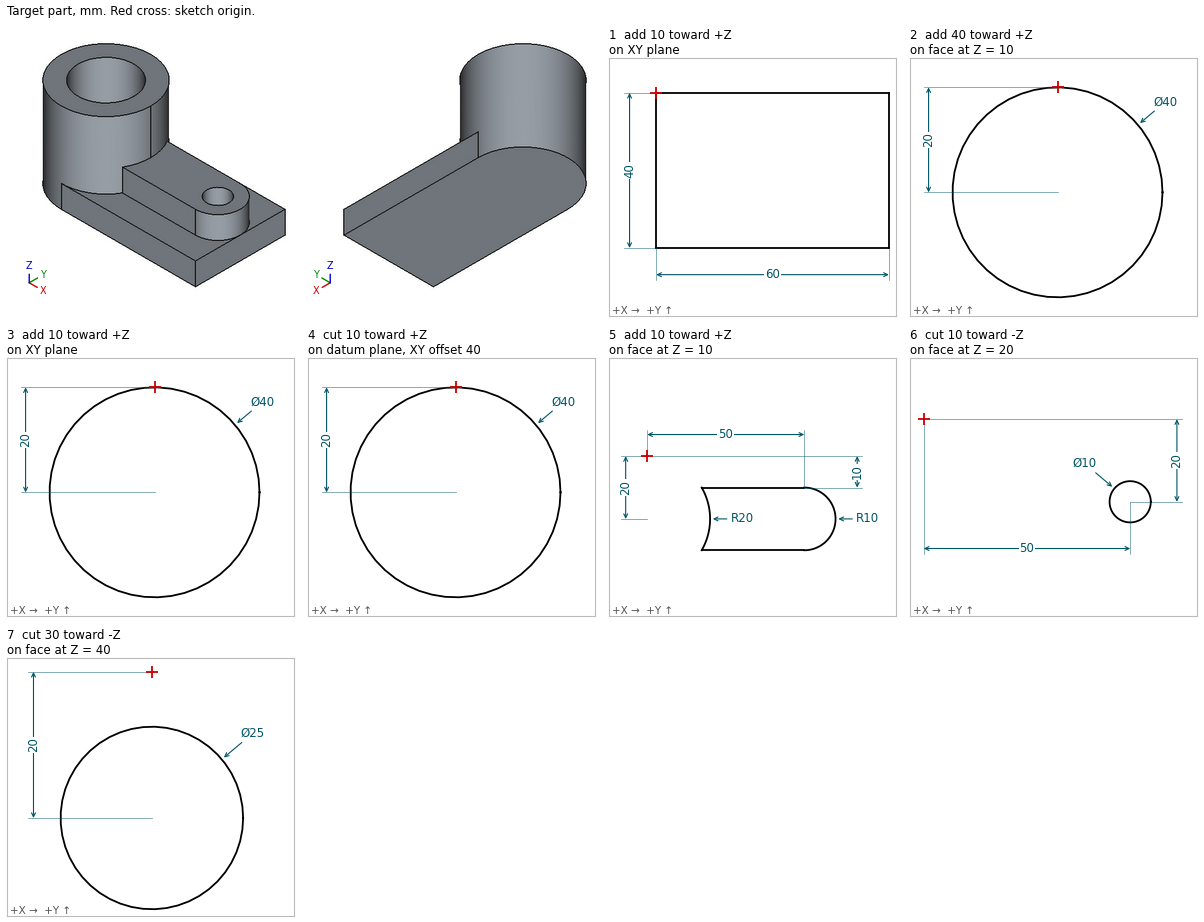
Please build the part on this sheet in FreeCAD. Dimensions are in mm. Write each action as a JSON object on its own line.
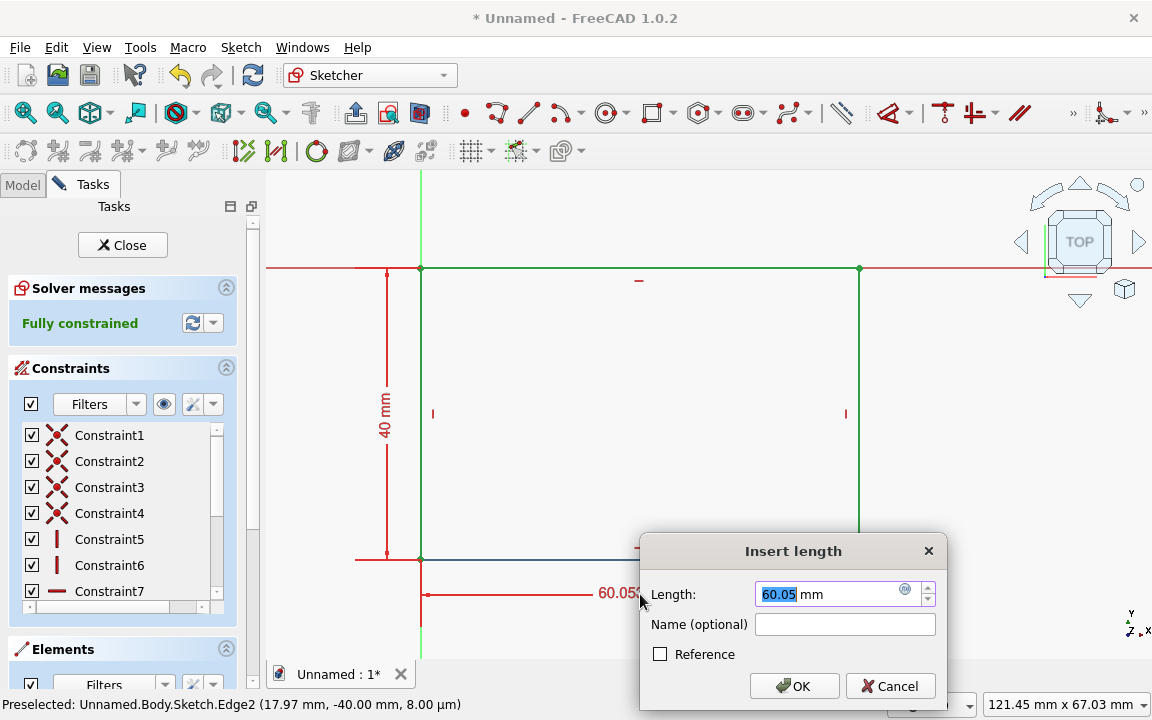
{"action": "type", "text": "60"}
{"action": "key", "text": "Return"}
{"action": "key", "text": "Escape"}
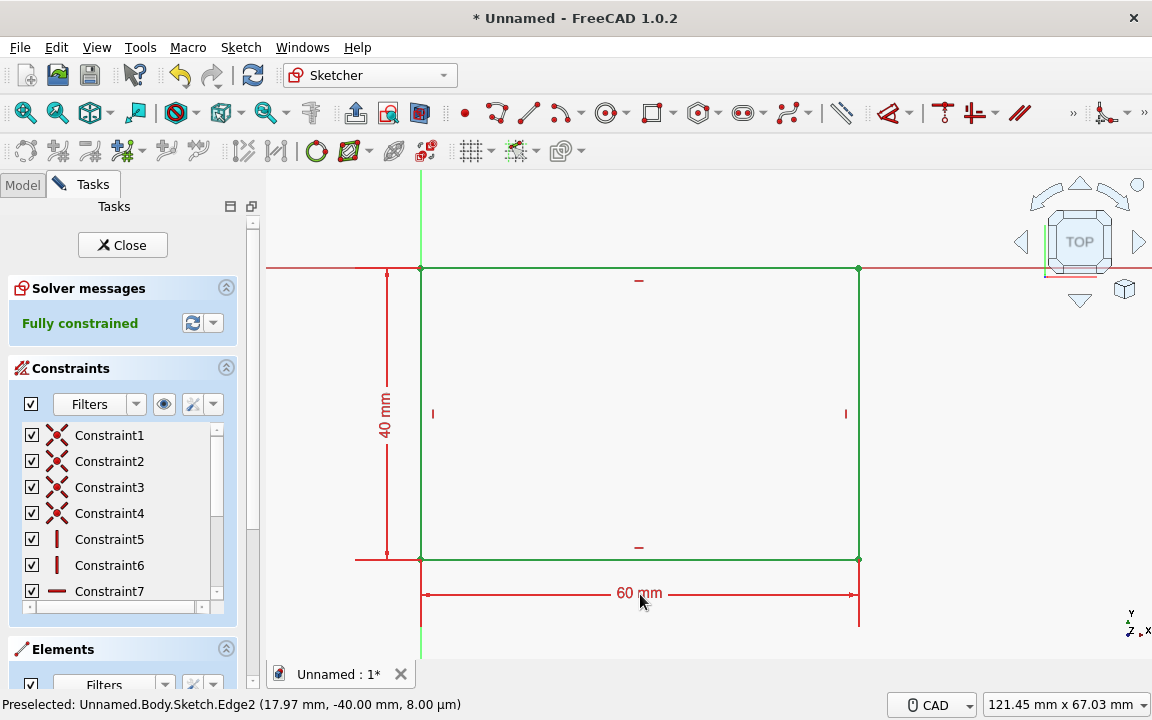
{"action": "left_click", "coordinate": [123, 245]}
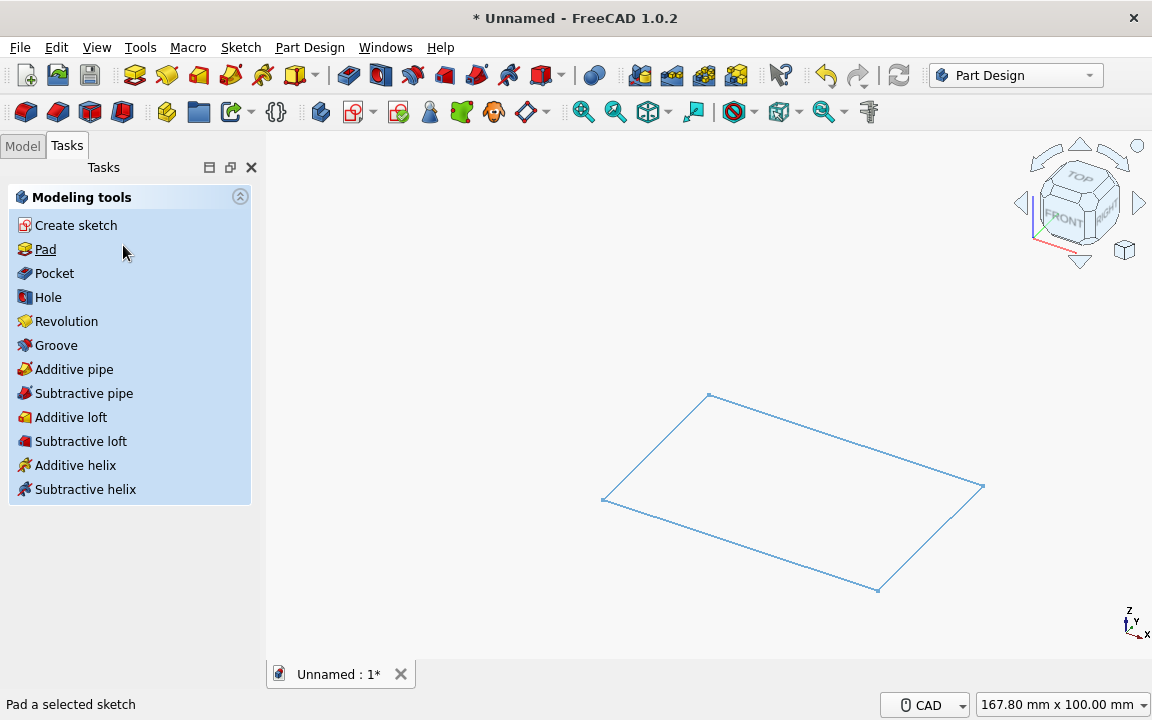
{"action": "left_click", "coordinate": [136, 76]}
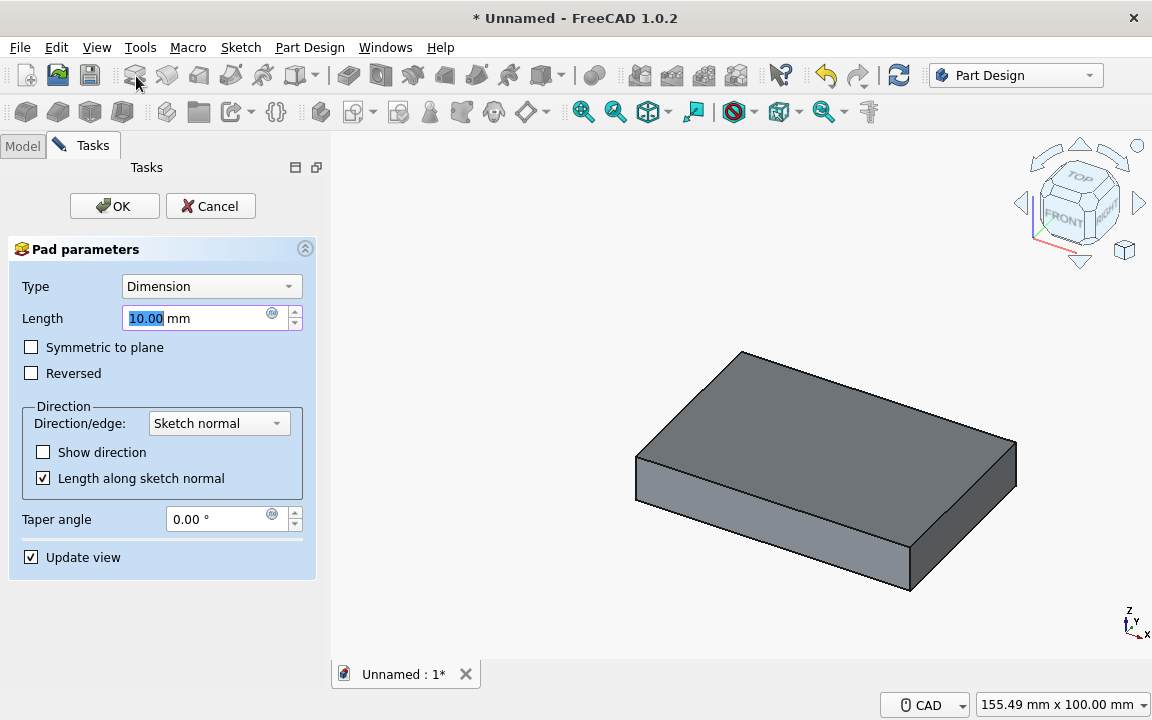
{"action": "type", "text": "10"}
{"action": "key", "text": "Tab"}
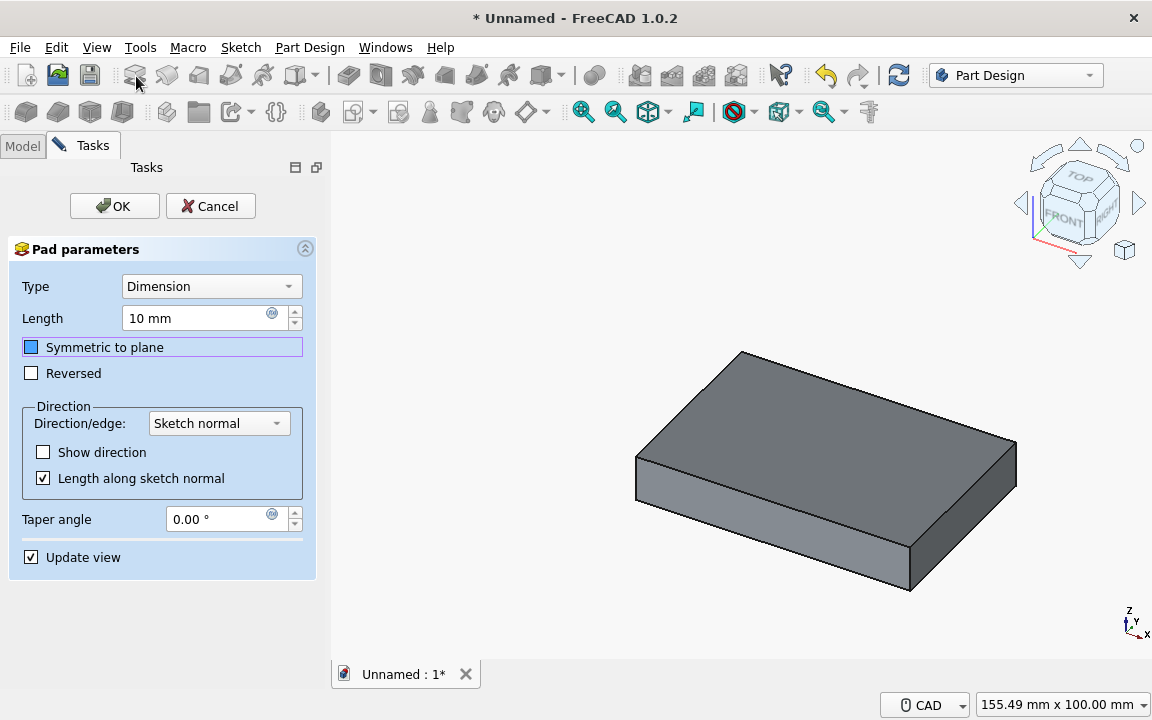
{"action": "left_click", "coordinate": [115, 206]}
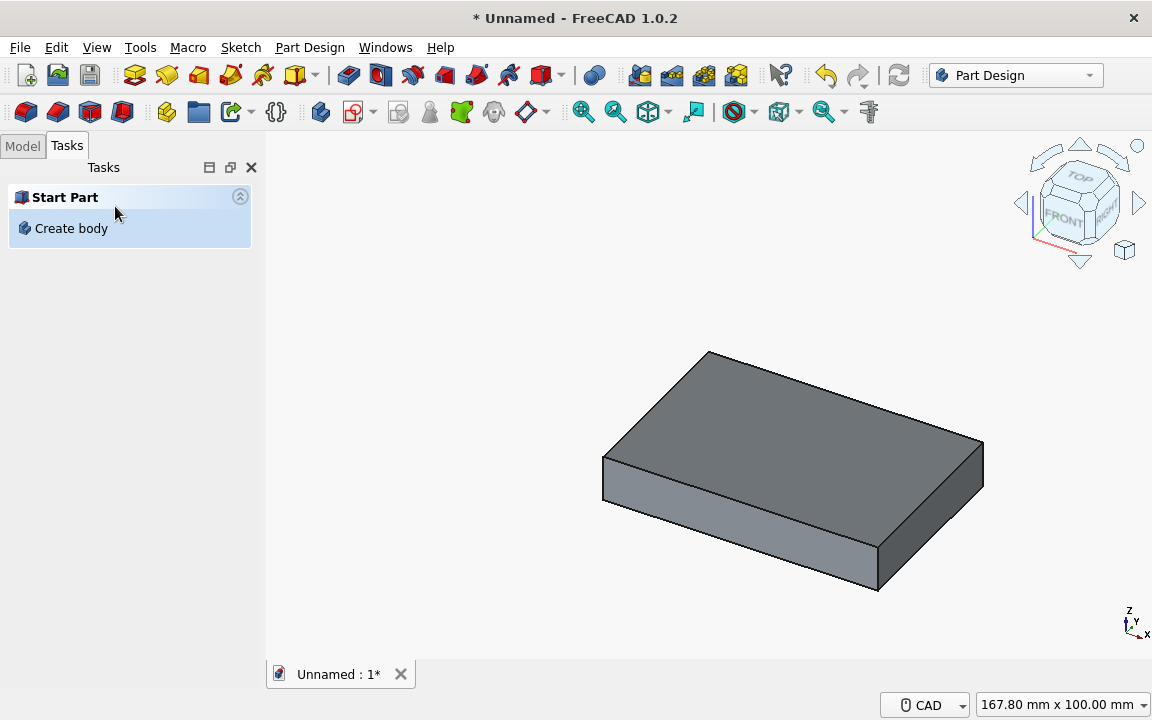
{"action": "left_click", "coordinate": [833, 462]}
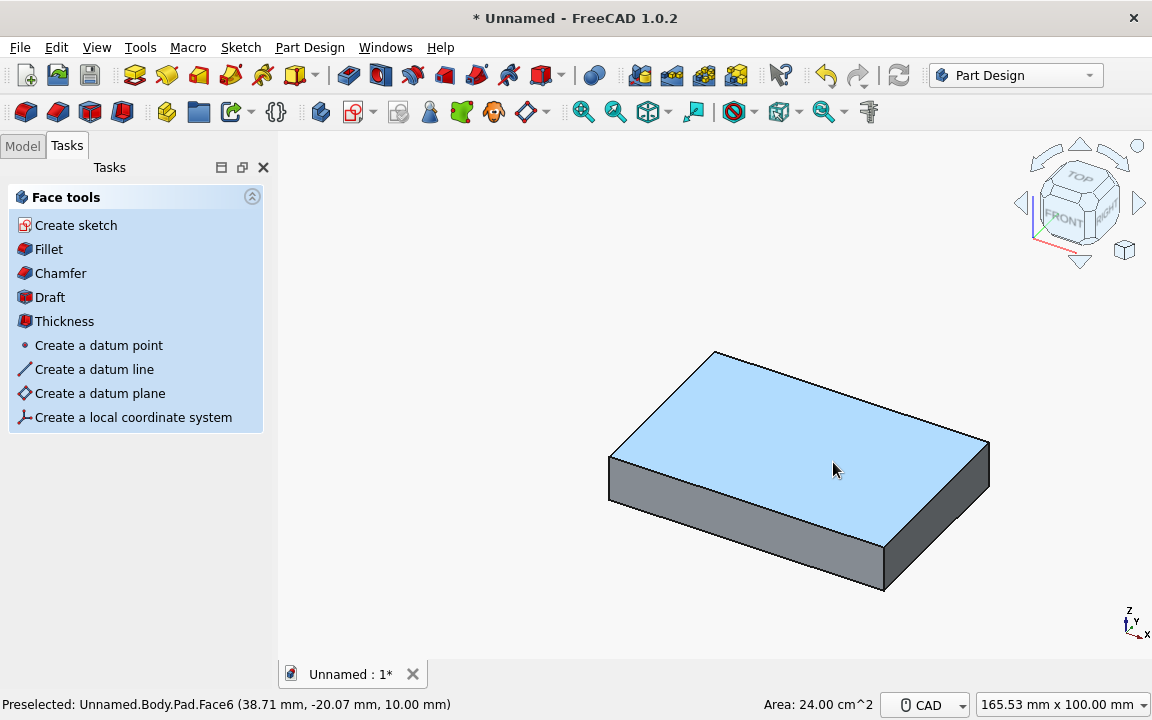
{"action": "left_click", "coordinate": [354, 112]}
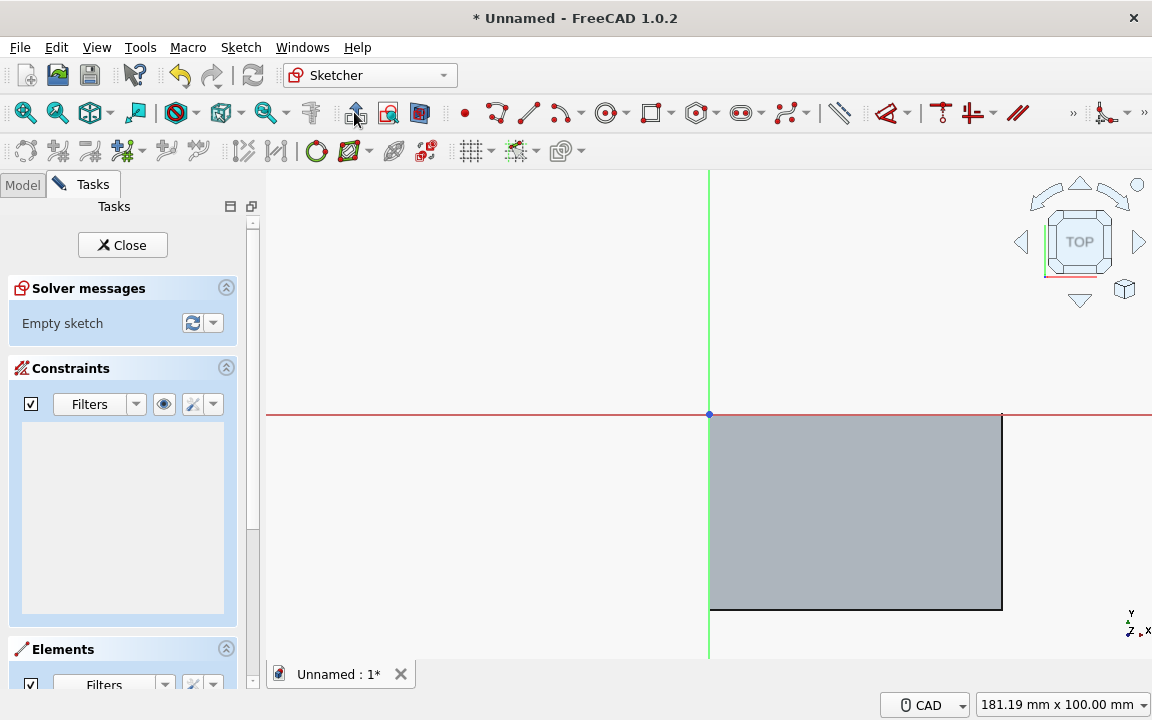
{"action": "scroll", "coordinate": [848, 631], "scroll_direction": "up", "scroll_amount": 2}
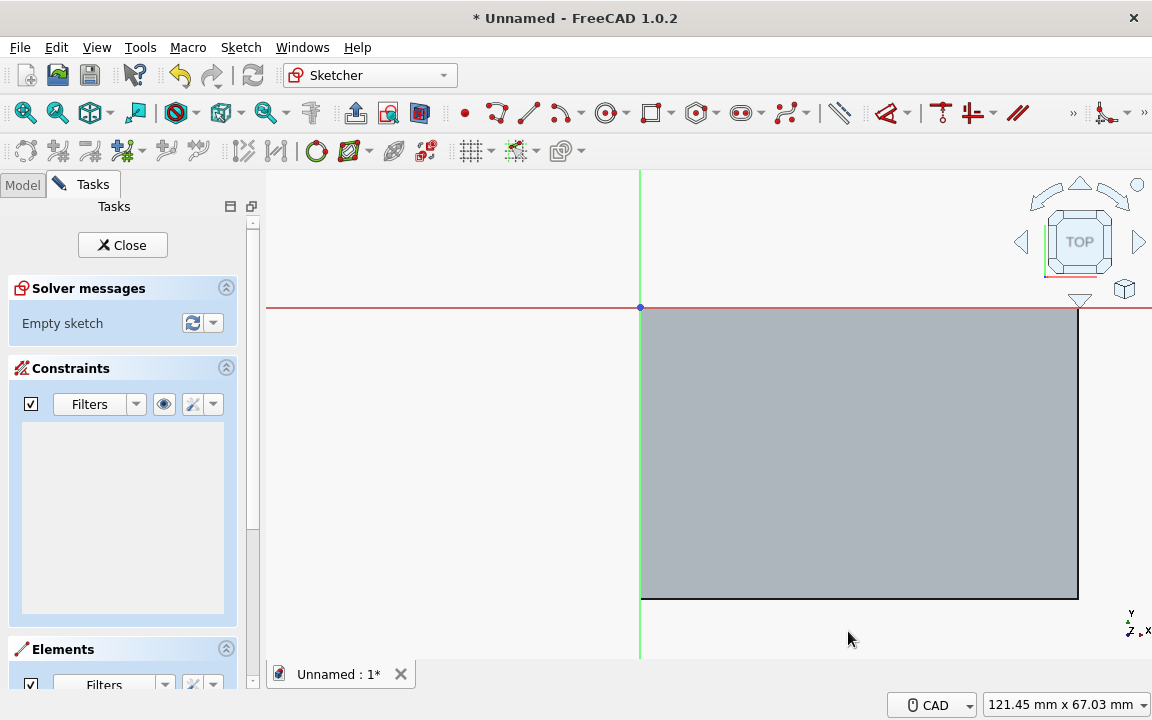
{"action": "left_click", "coordinate": [606, 114]}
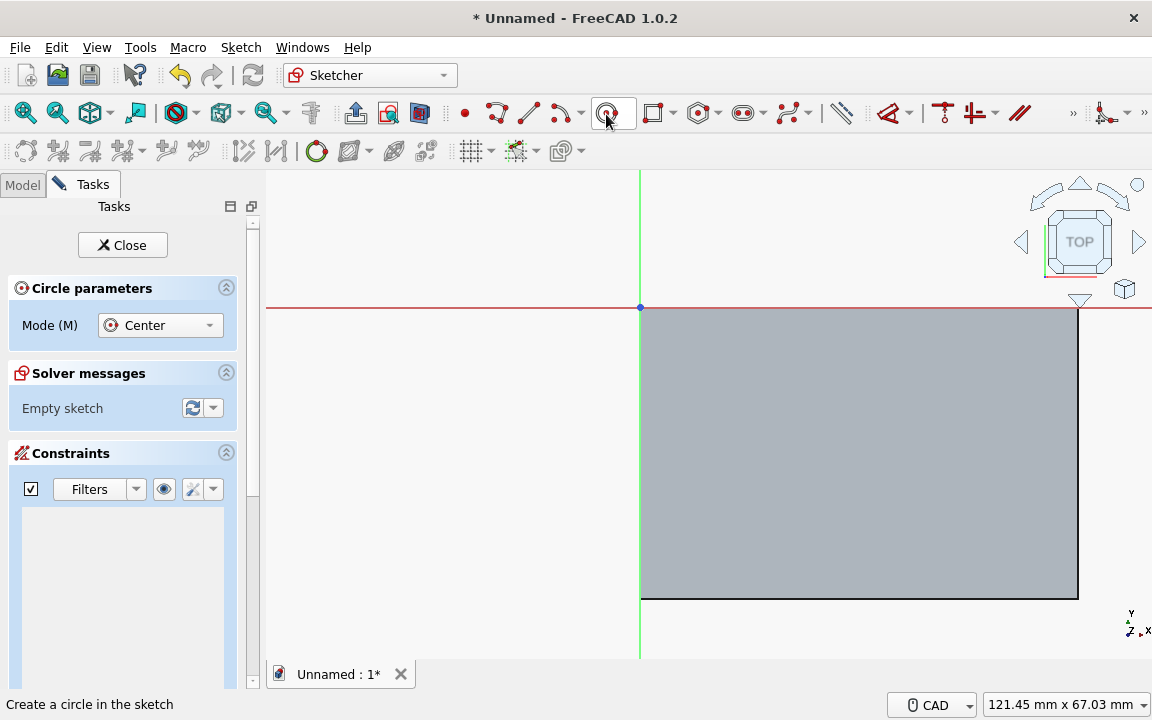
{"action": "left_click", "coordinate": [640, 453]}
{"action": "left_click", "coordinate": [743, 350]}
{"action": "key", "text": "Escape"}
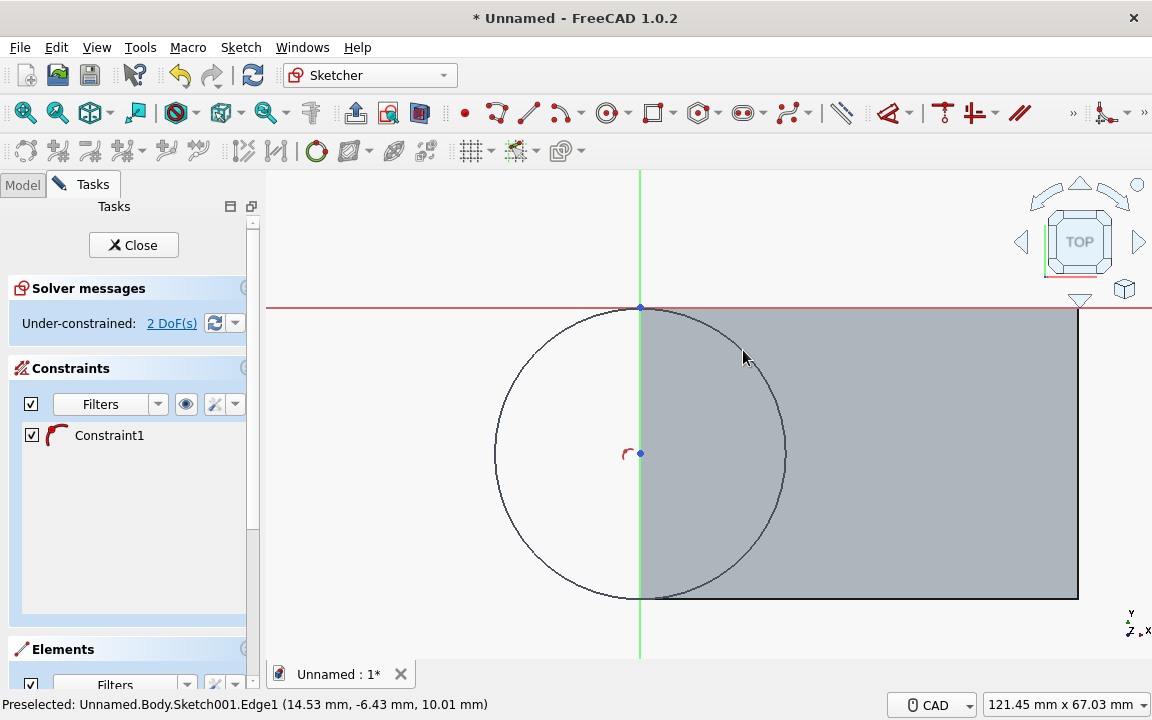
{"action": "left_click", "coordinate": [888, 114]}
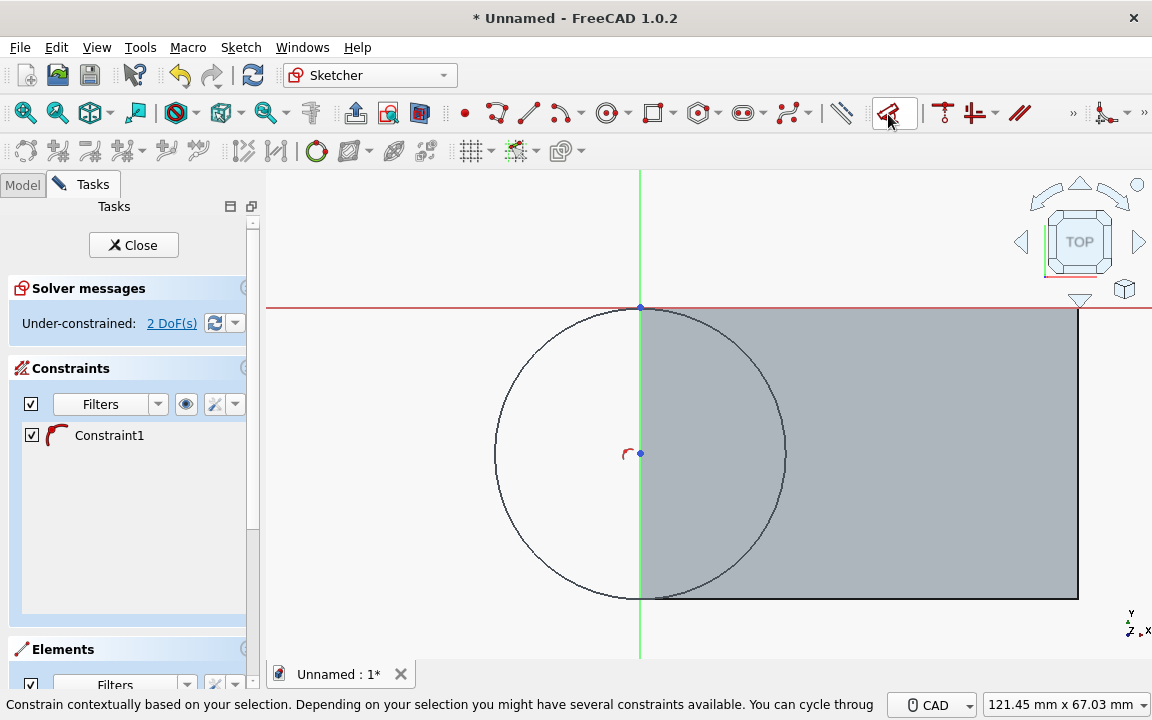
{"action": "left_click", "coordinate": [743, 351]}
{"action": "left_click", "coordinate": [766, 328]}